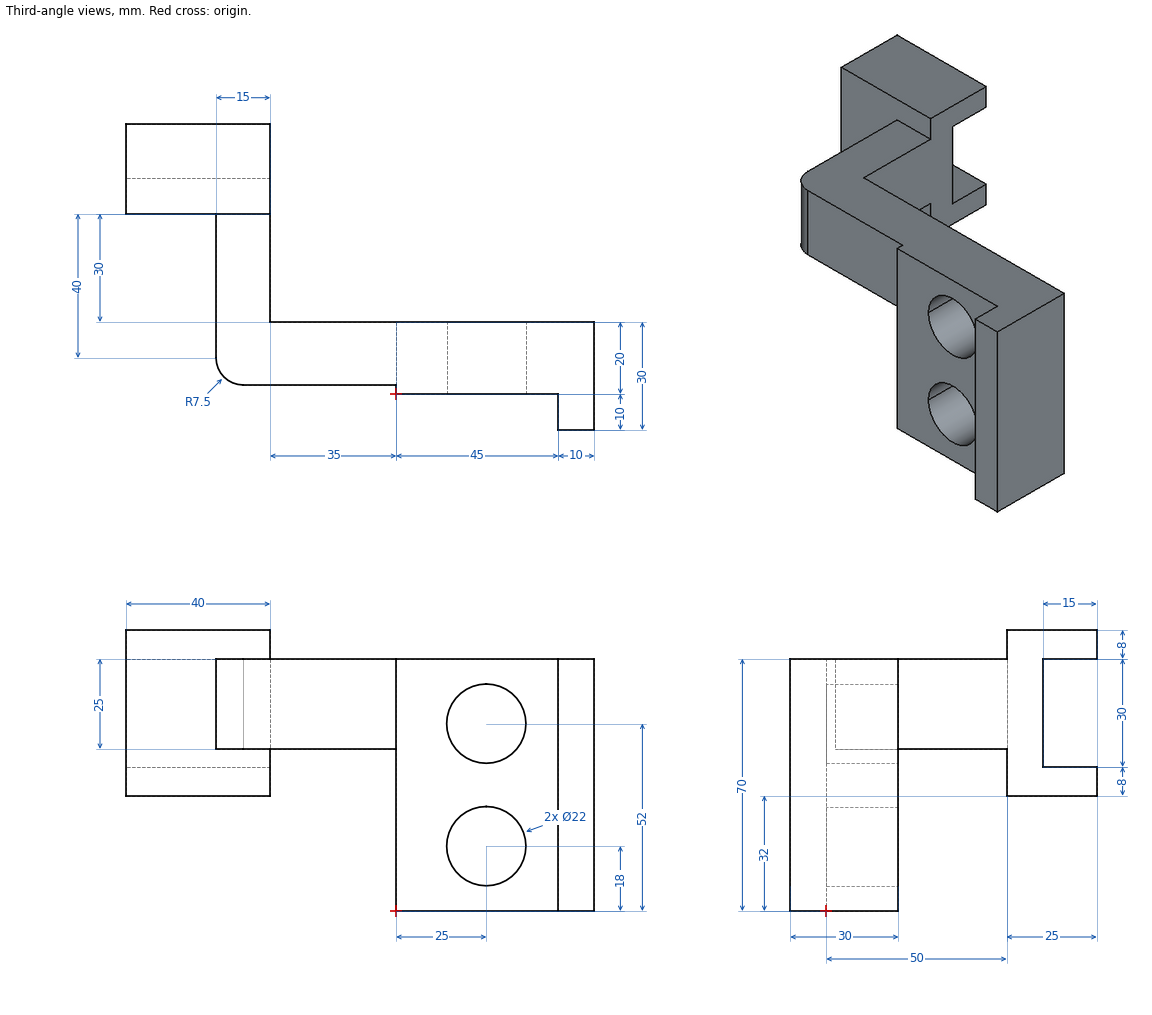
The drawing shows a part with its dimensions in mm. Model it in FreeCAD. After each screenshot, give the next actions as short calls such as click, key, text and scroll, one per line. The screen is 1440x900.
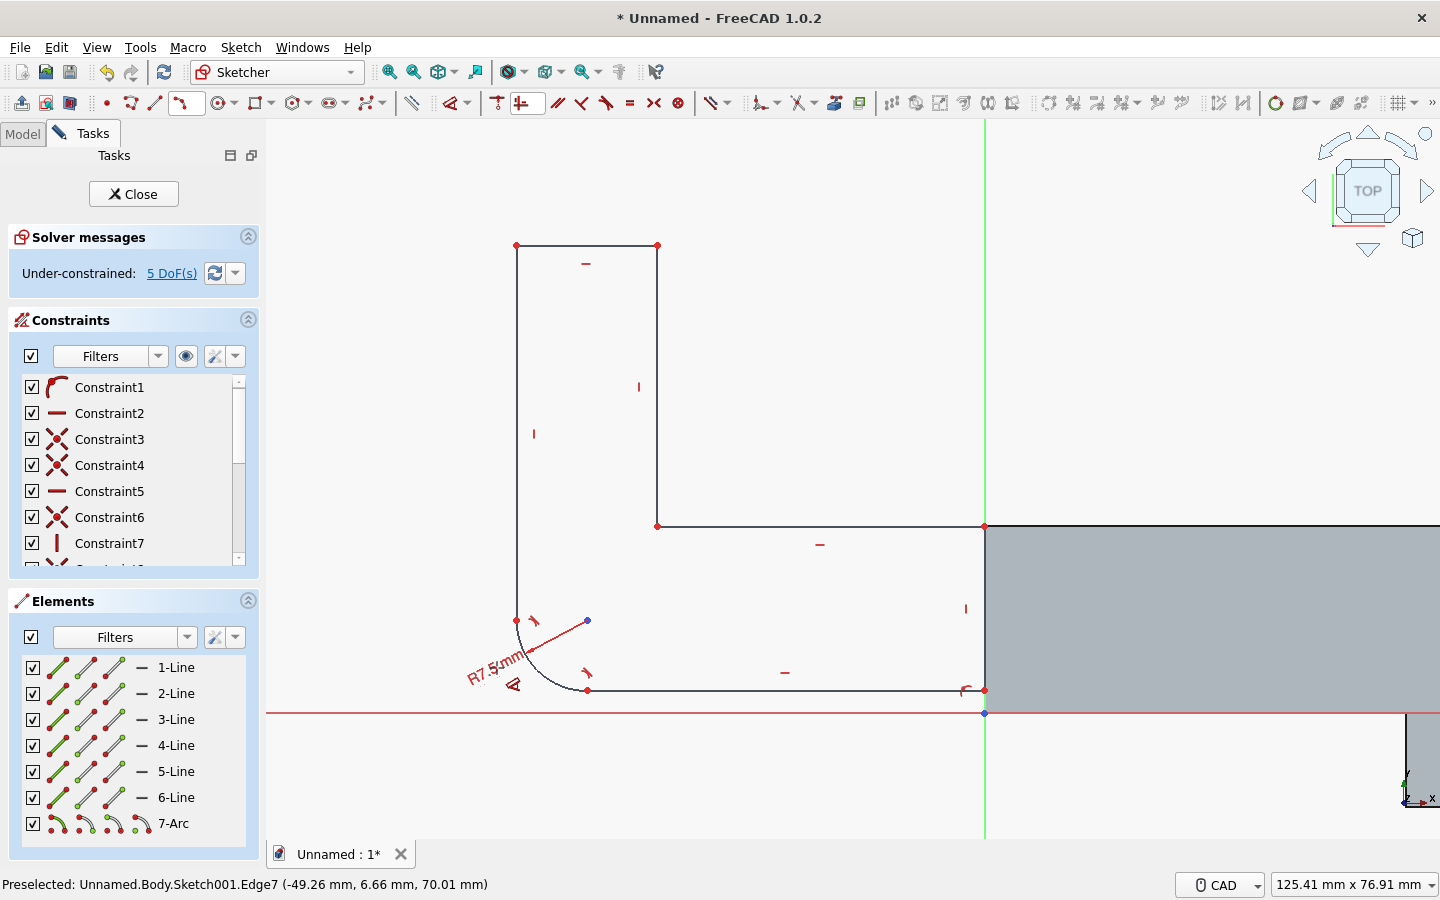
click(886, 527)
click(821, 561)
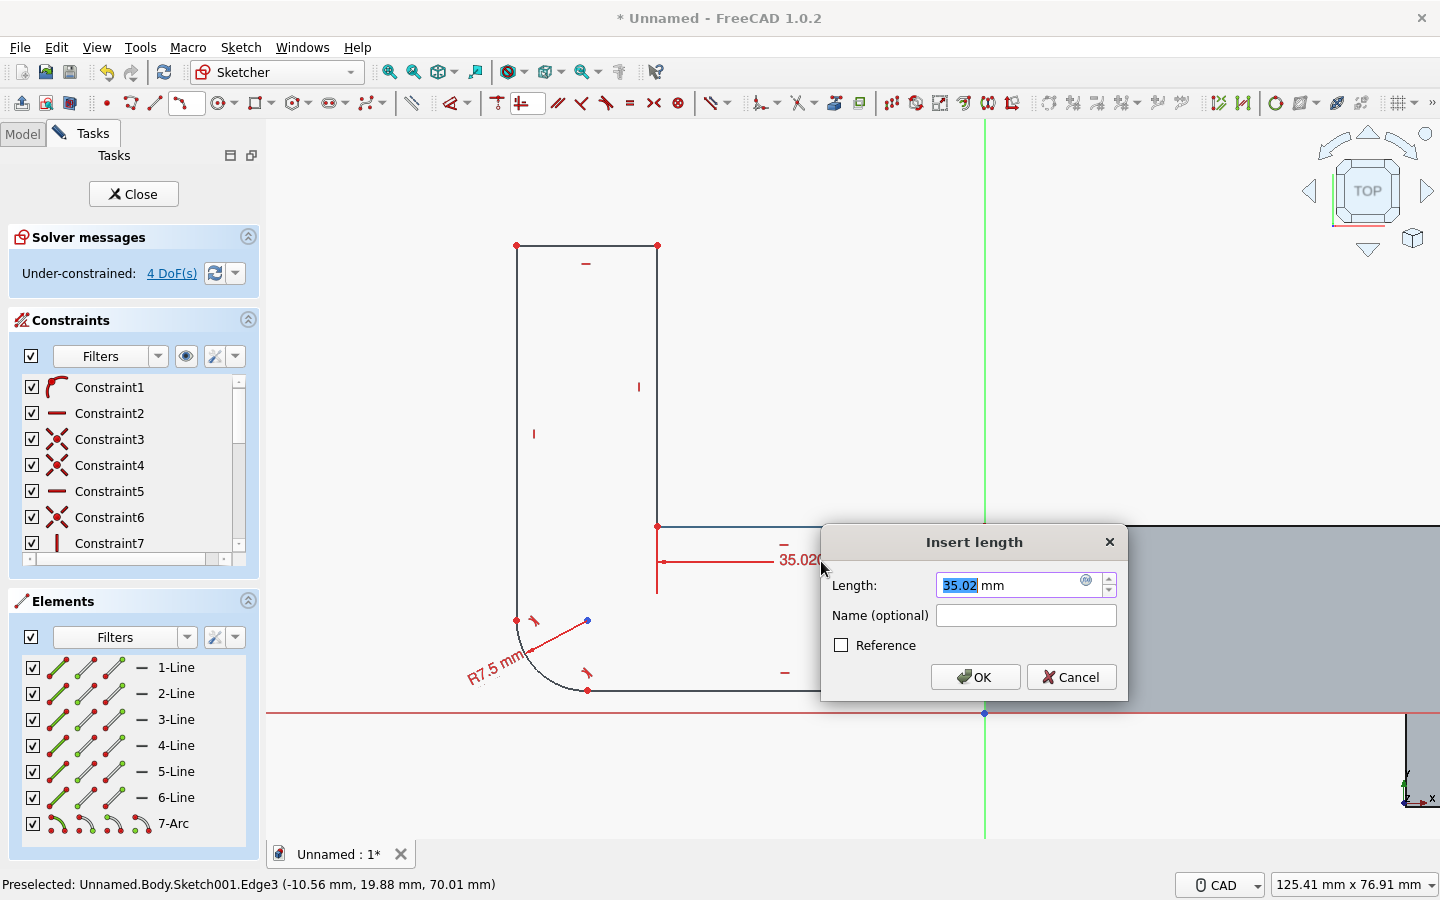
text(35)
key(Return)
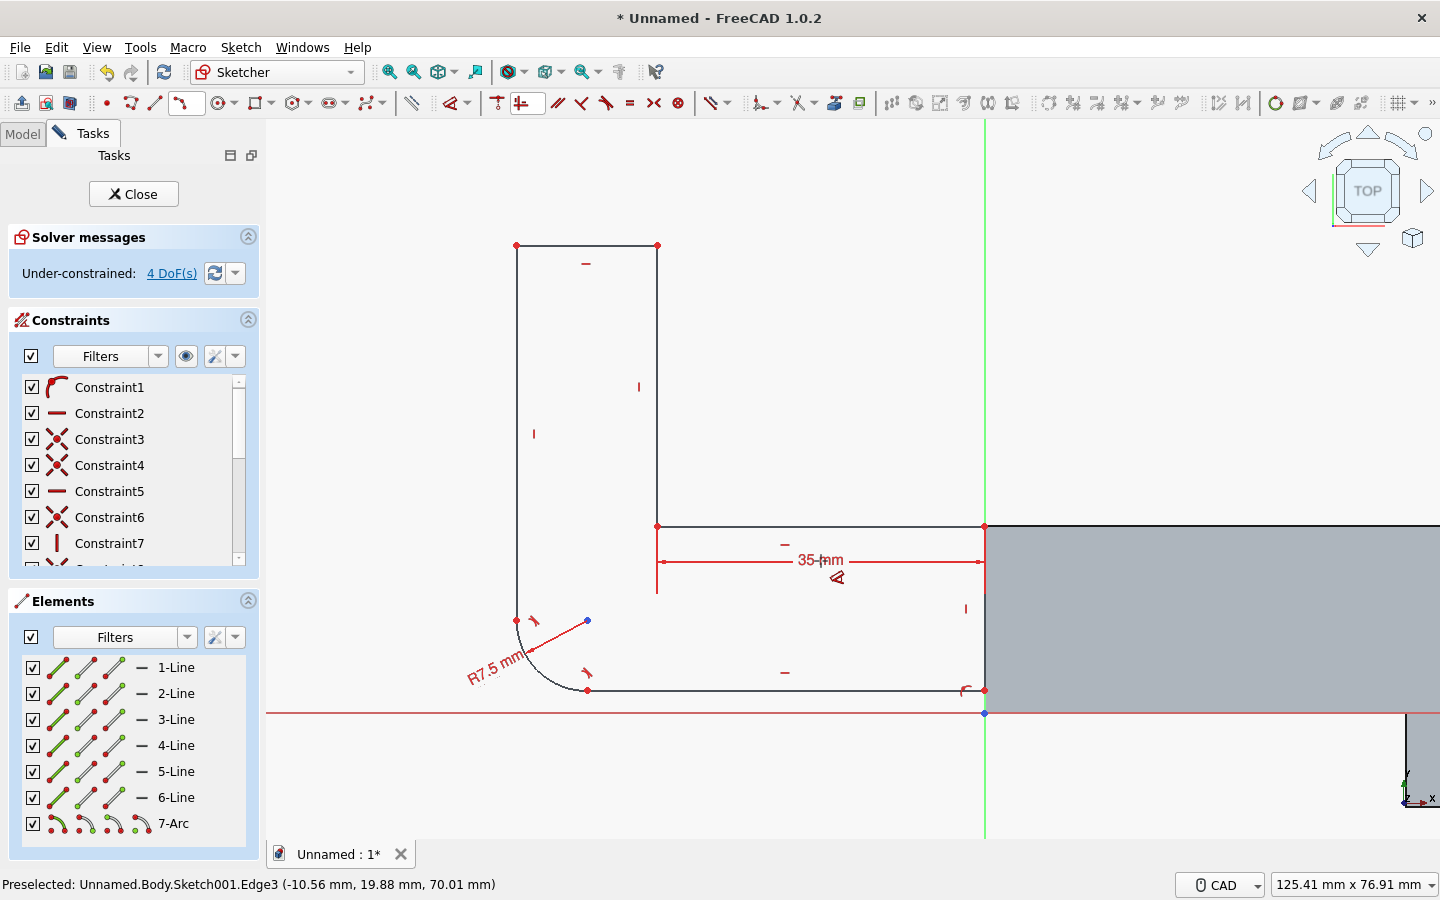
click(657, 443)
click(623, 386)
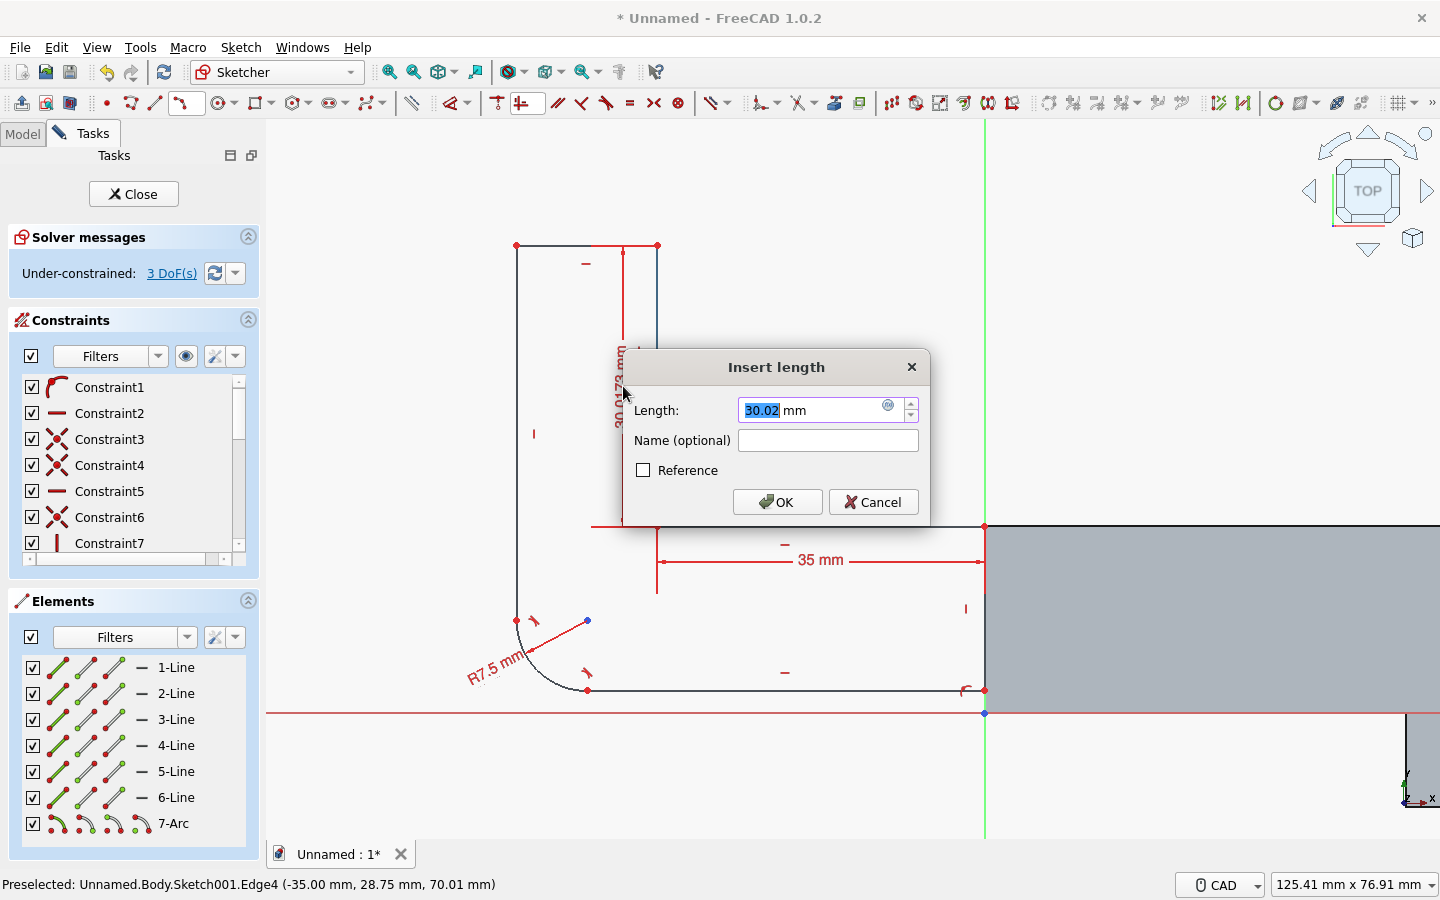
text(30)
key(Return)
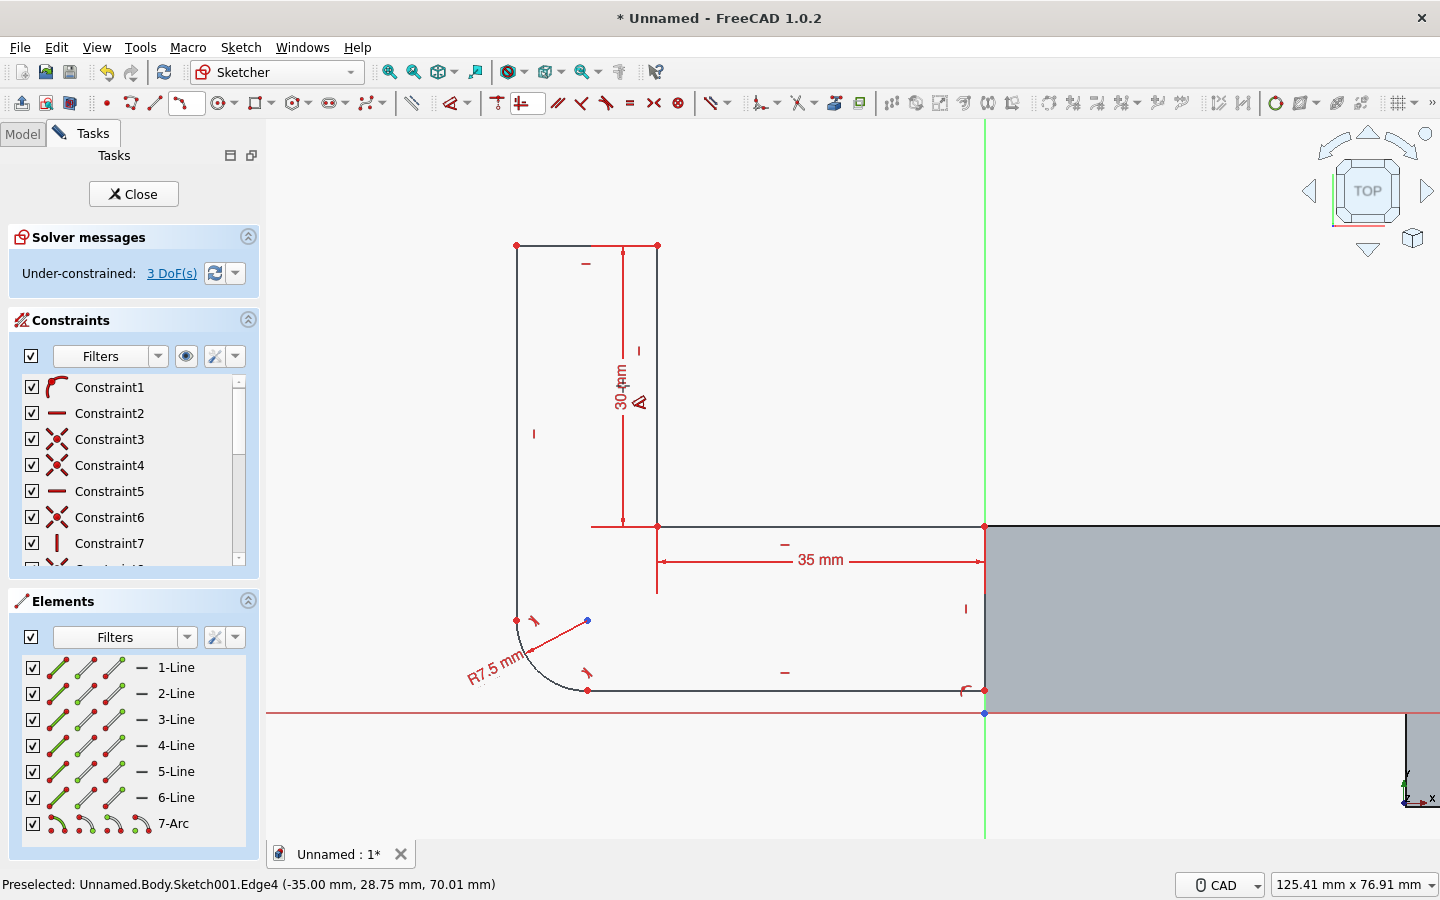
click(615, 246)
click(587, 212)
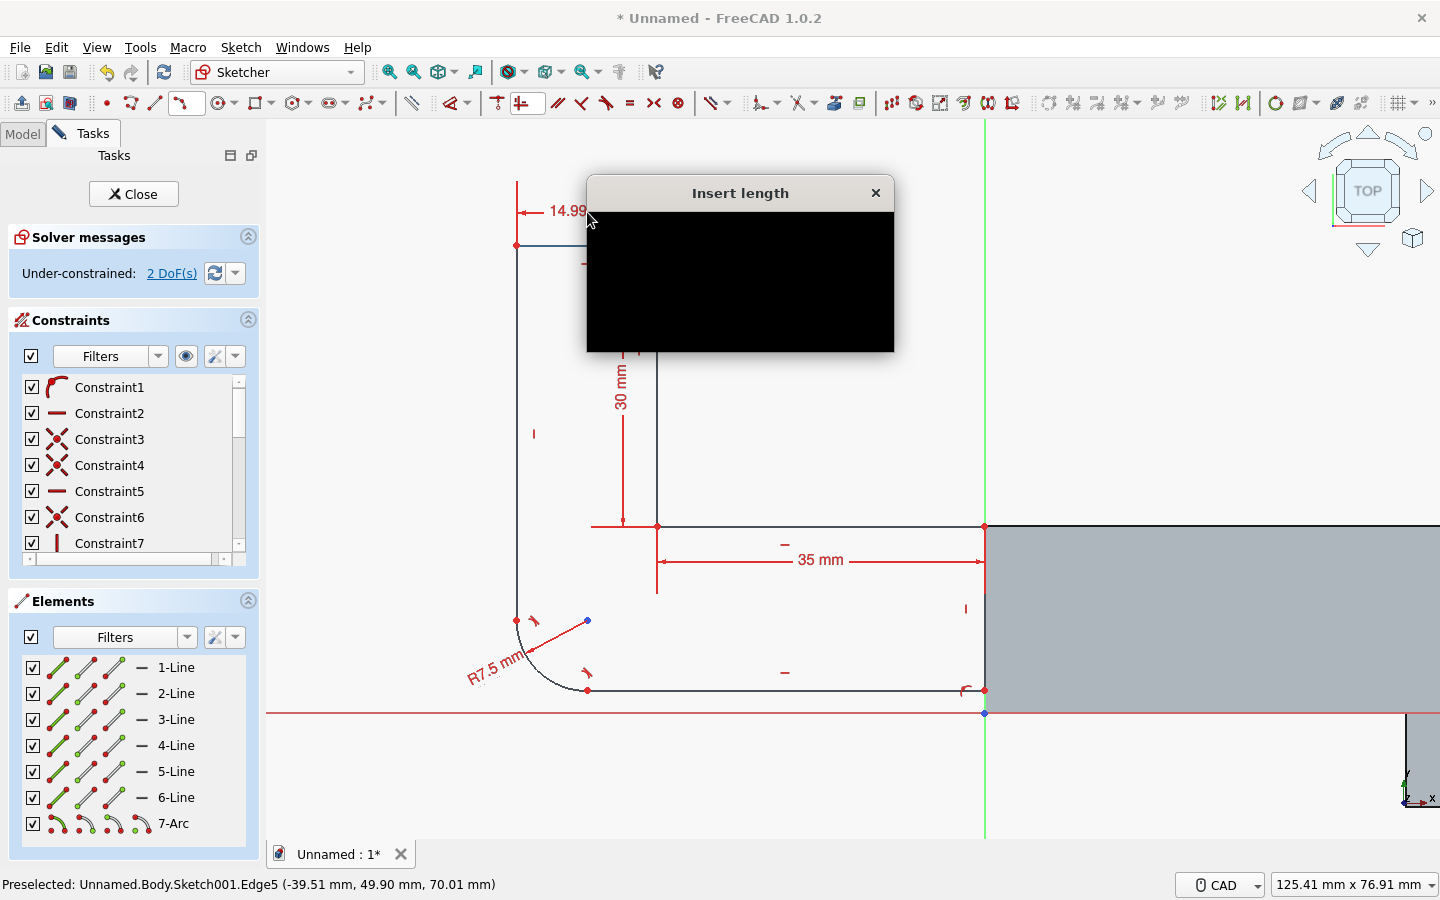
text(15)
key(Return)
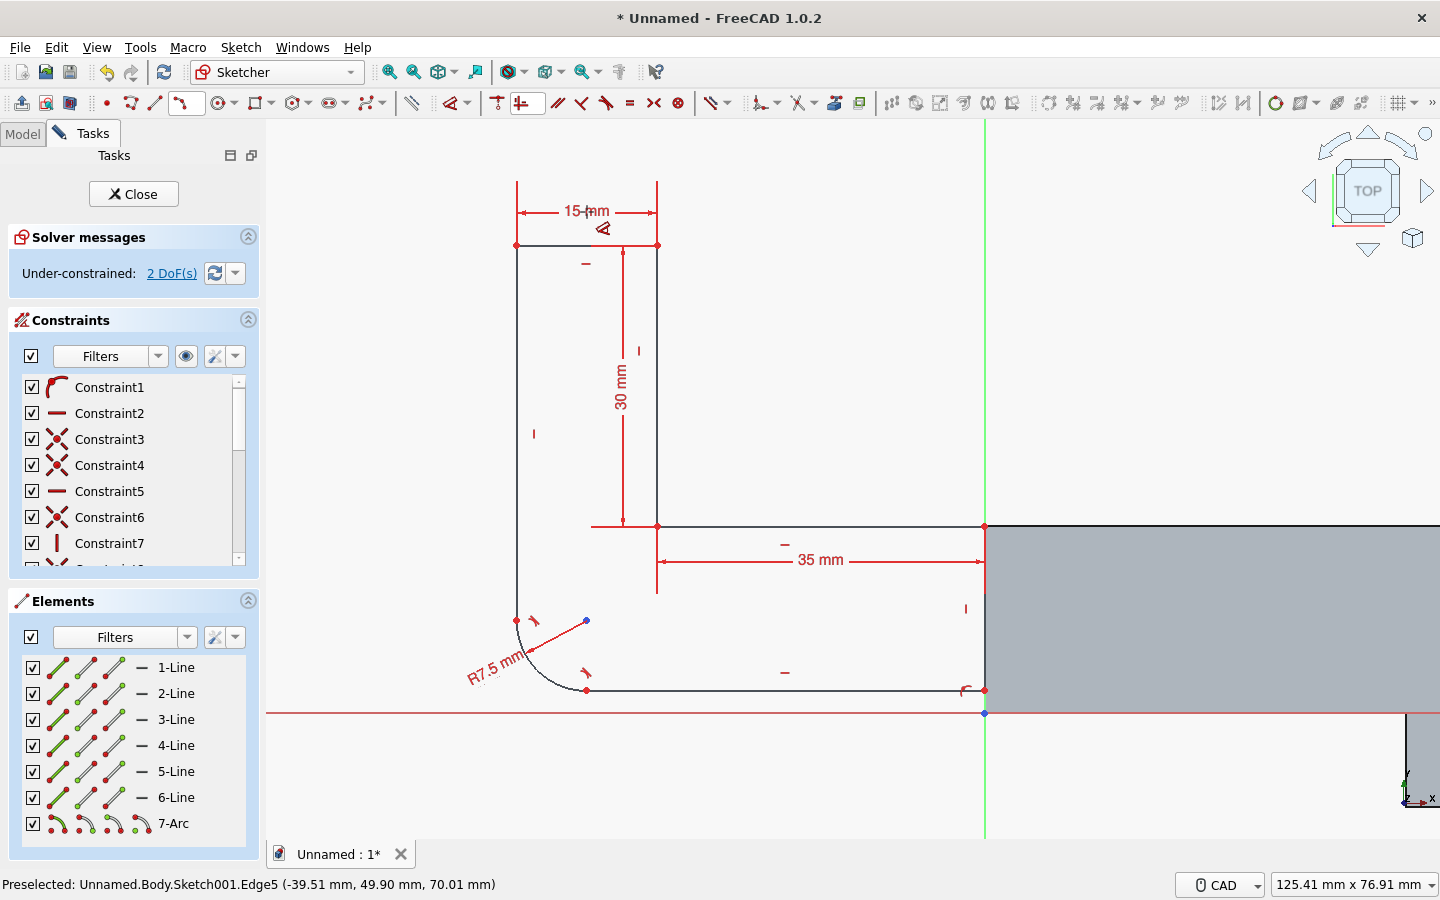
click(517, 358)
click(483, 433)